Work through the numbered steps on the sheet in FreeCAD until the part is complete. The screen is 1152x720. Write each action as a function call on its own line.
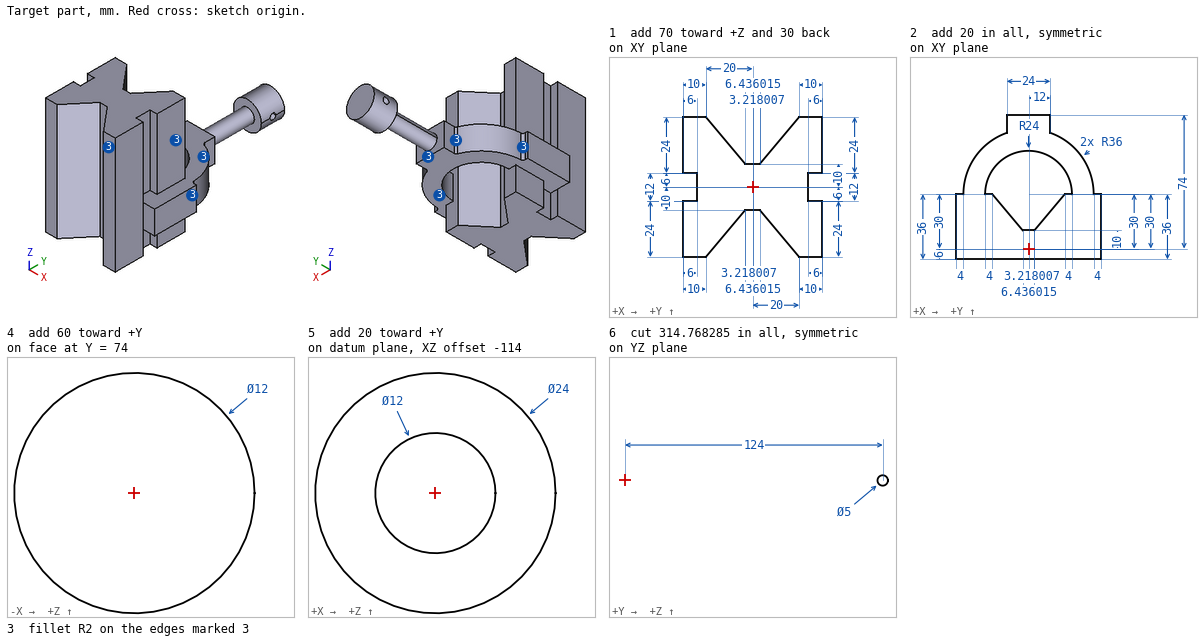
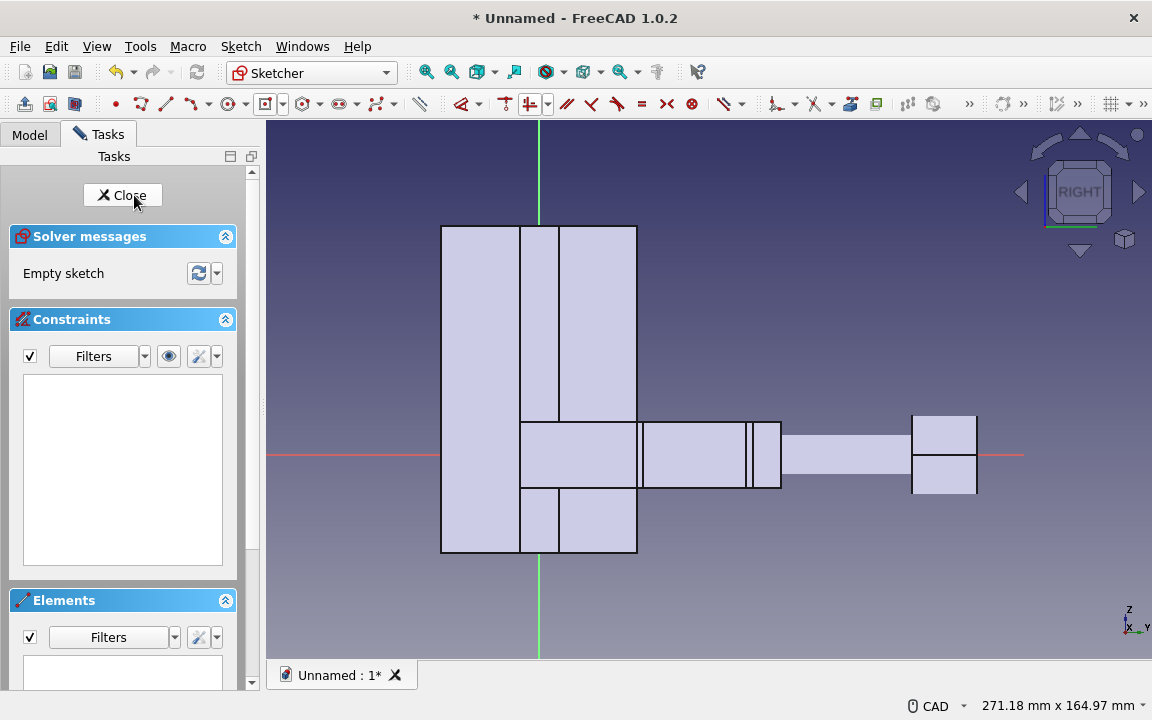
click(75, 104)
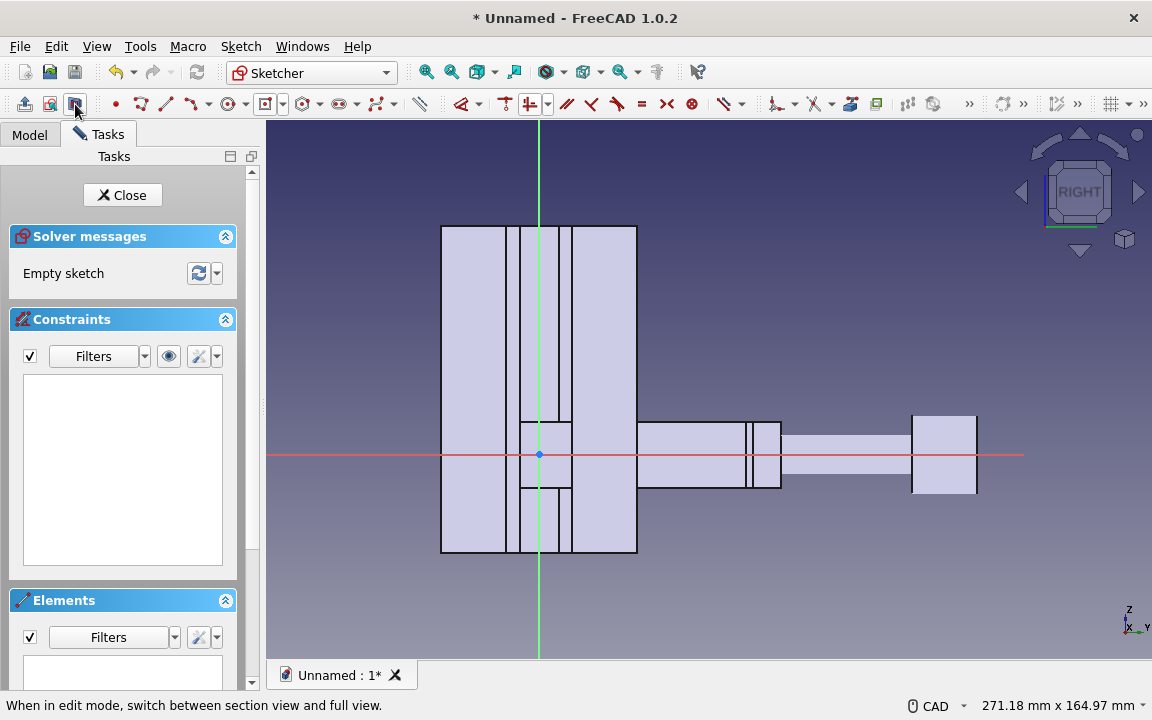
scroll(960, 458, up, 15)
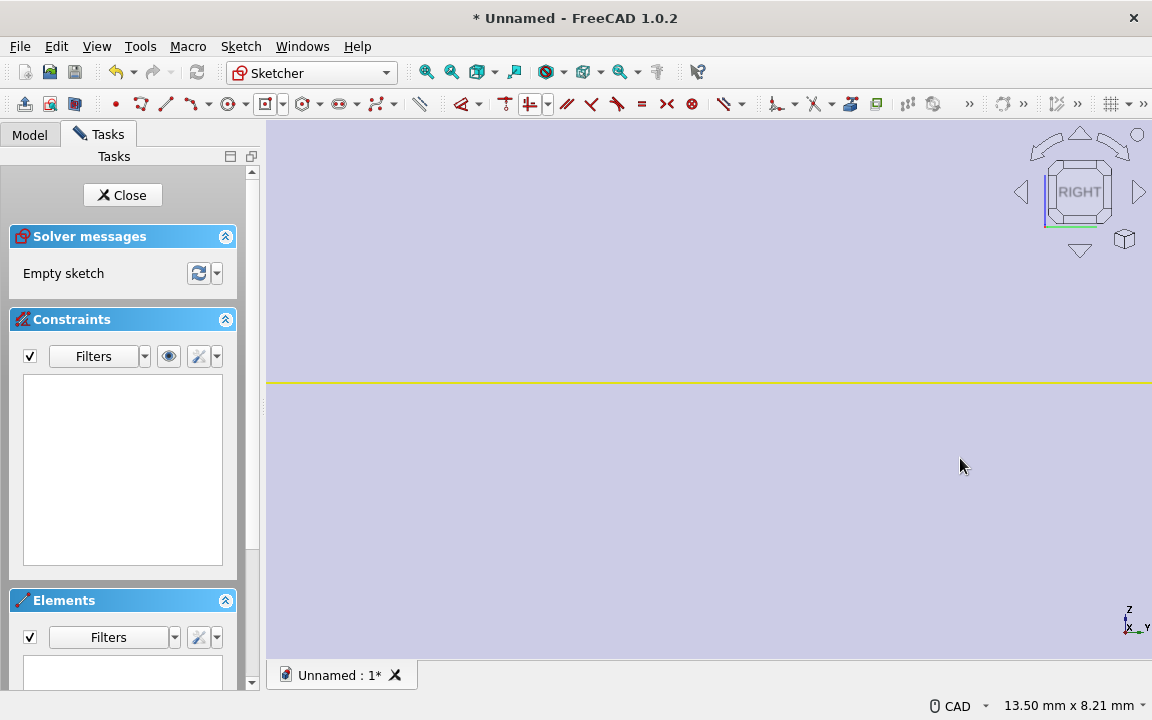
click(228, 104)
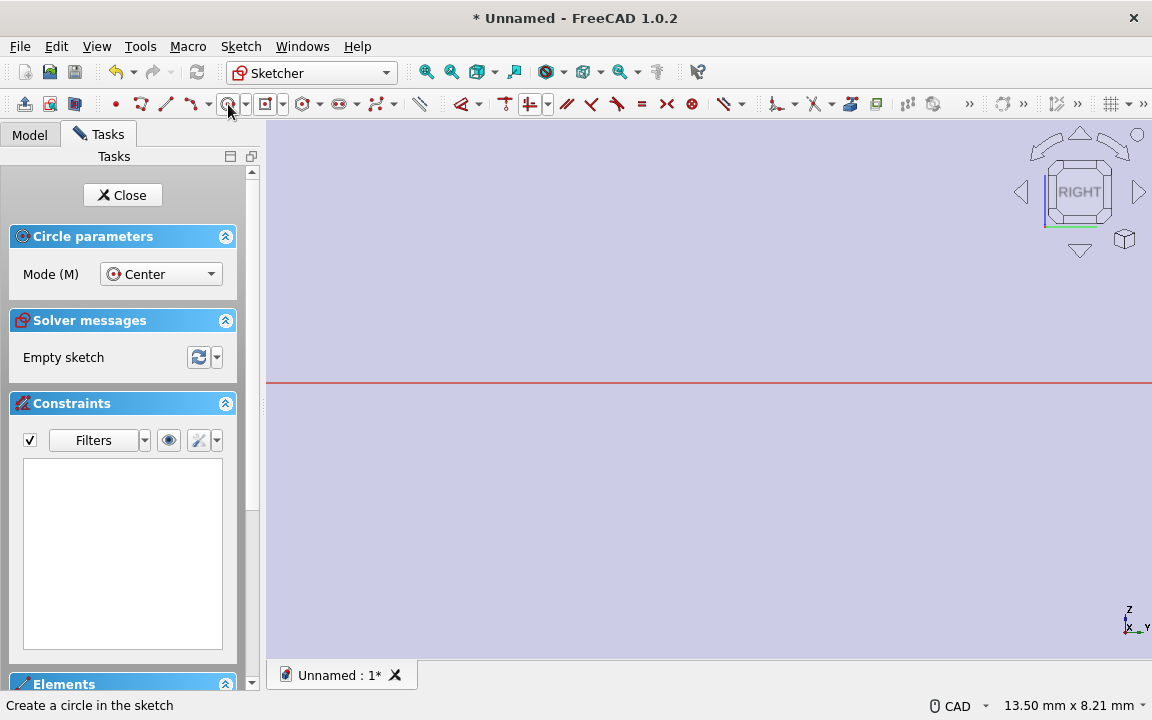
click(628, 383)
move(744, 267)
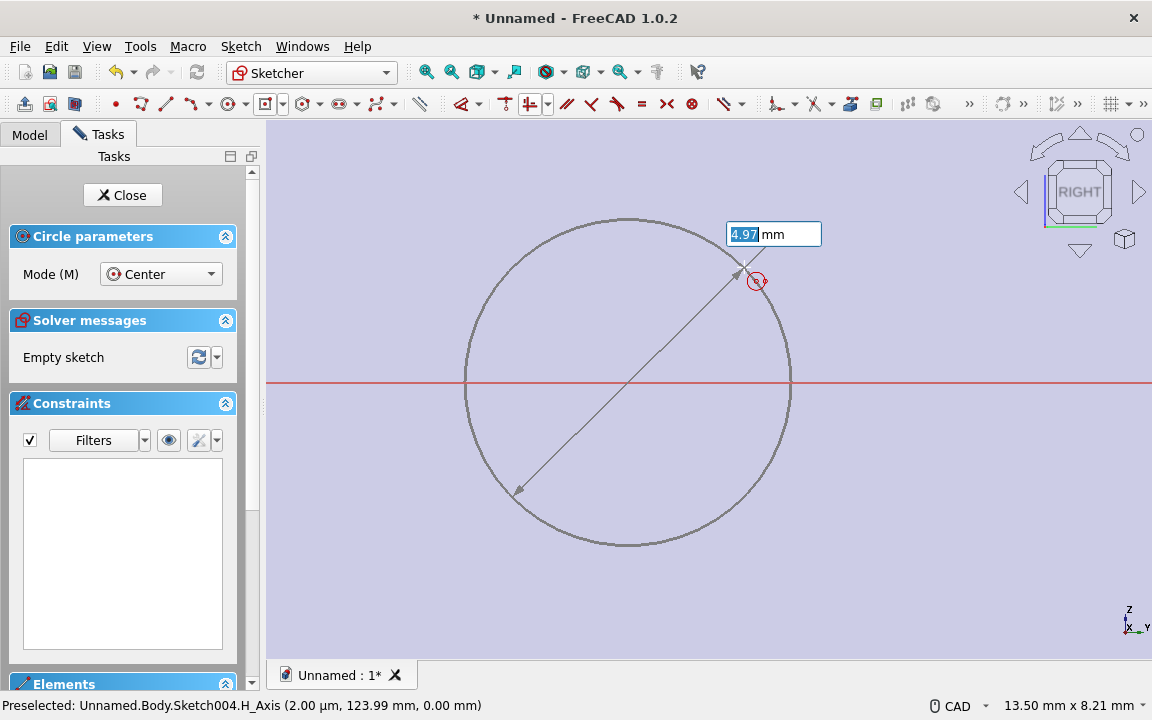
text(5)
key(Return)
key(Escape)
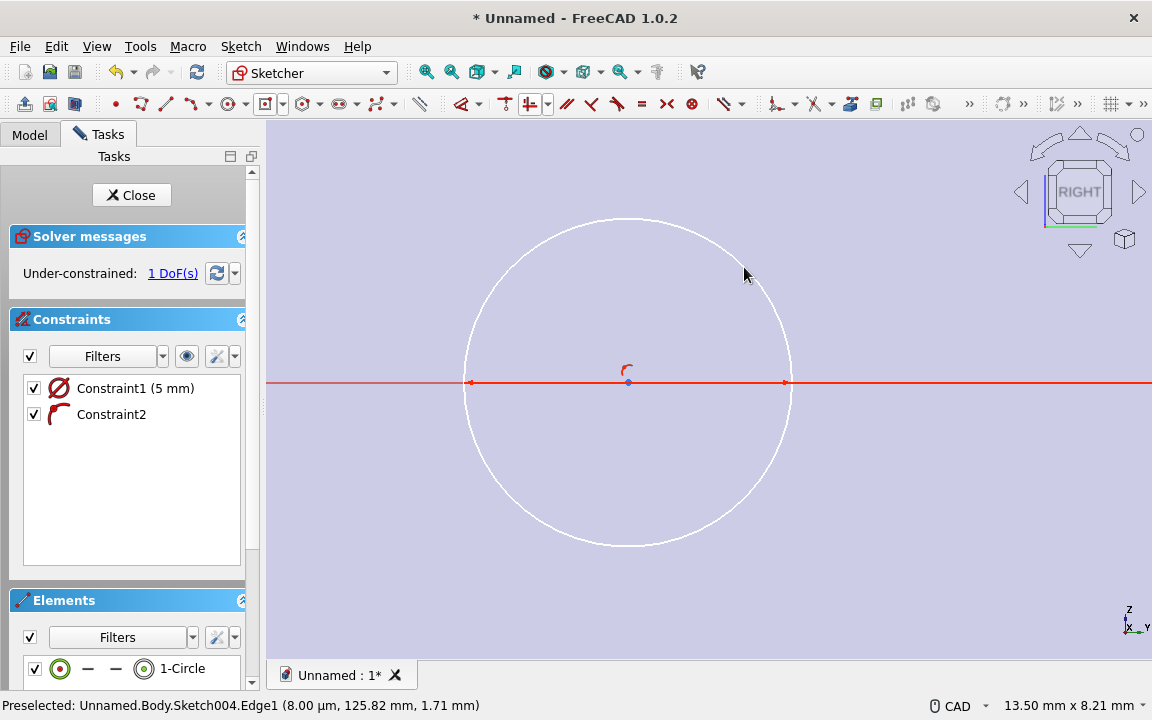
click(460, 104)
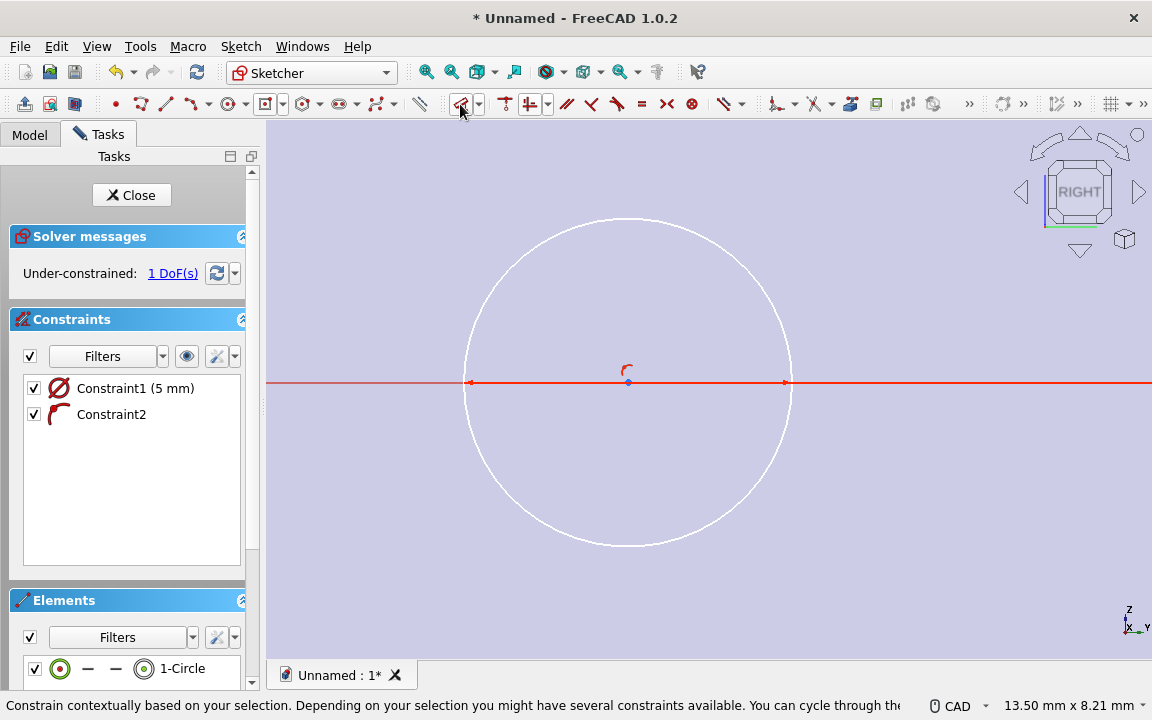
click(628, 383)
click(384, 417)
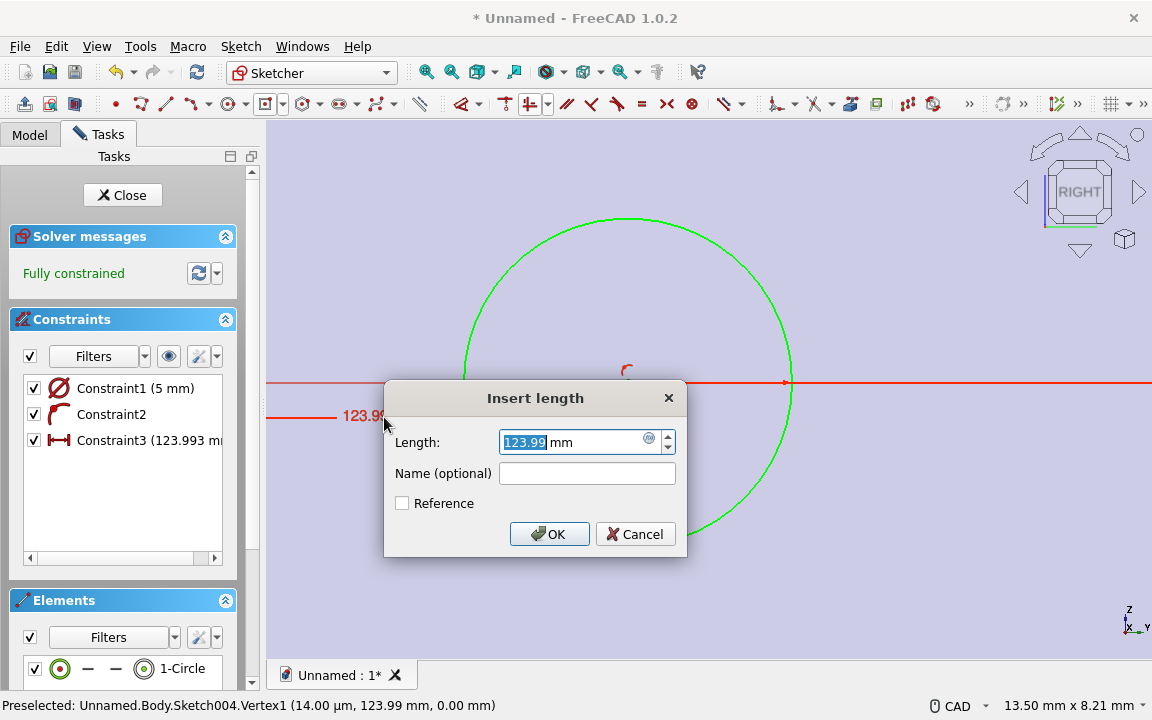
text(124)
key(Return)
key(Escape)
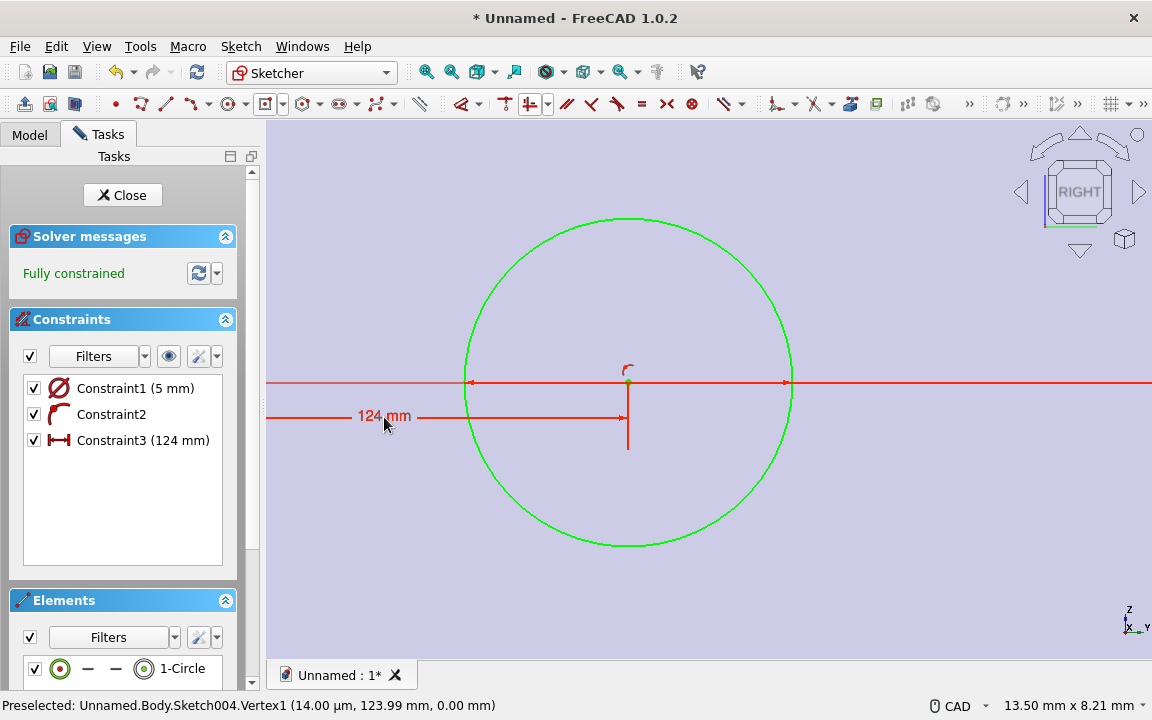
click(123, 195)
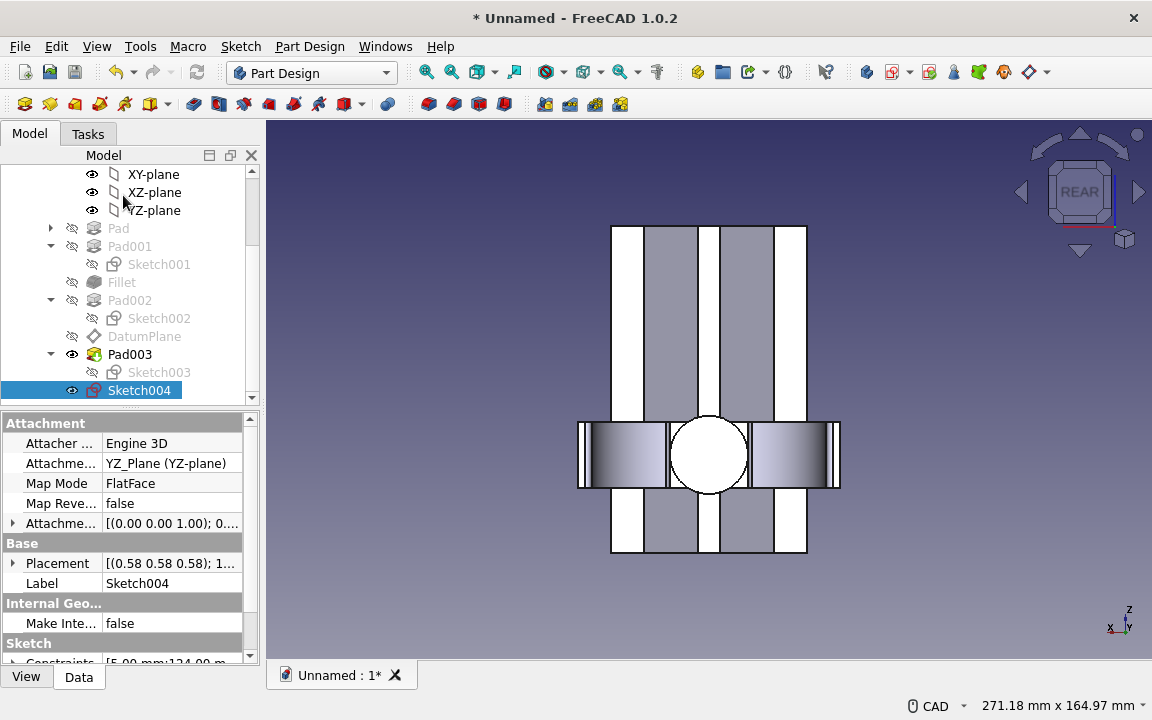
click(194, 104)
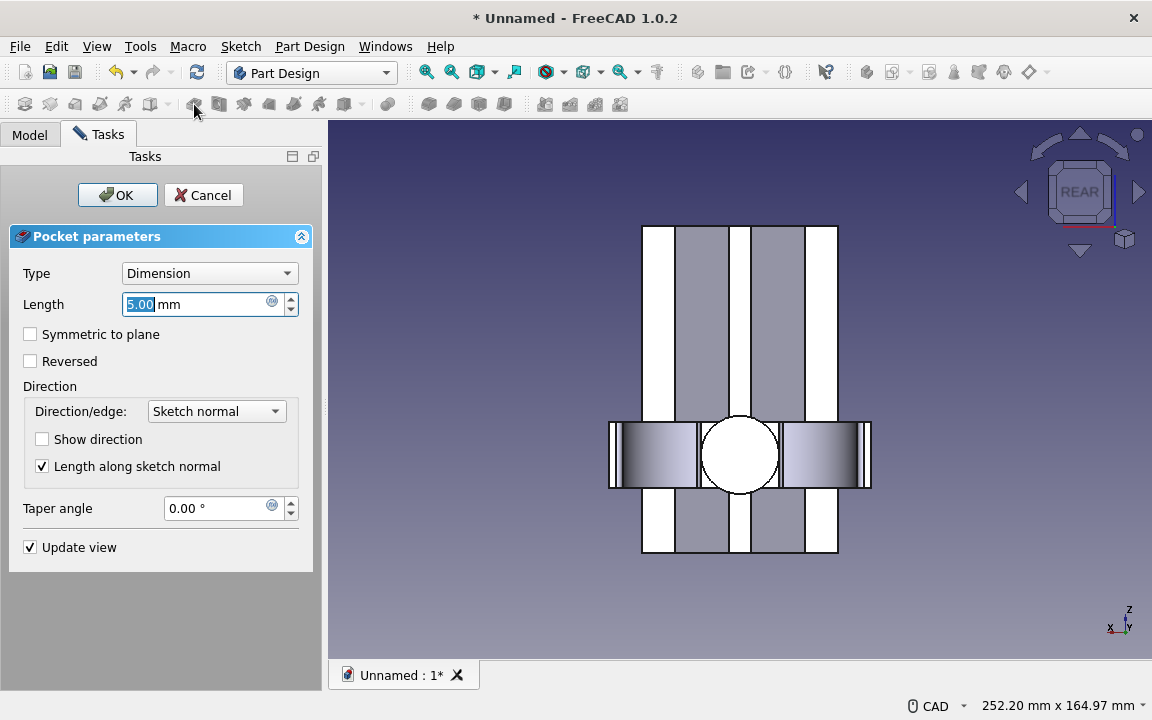
text(314.768285)
key(Tab)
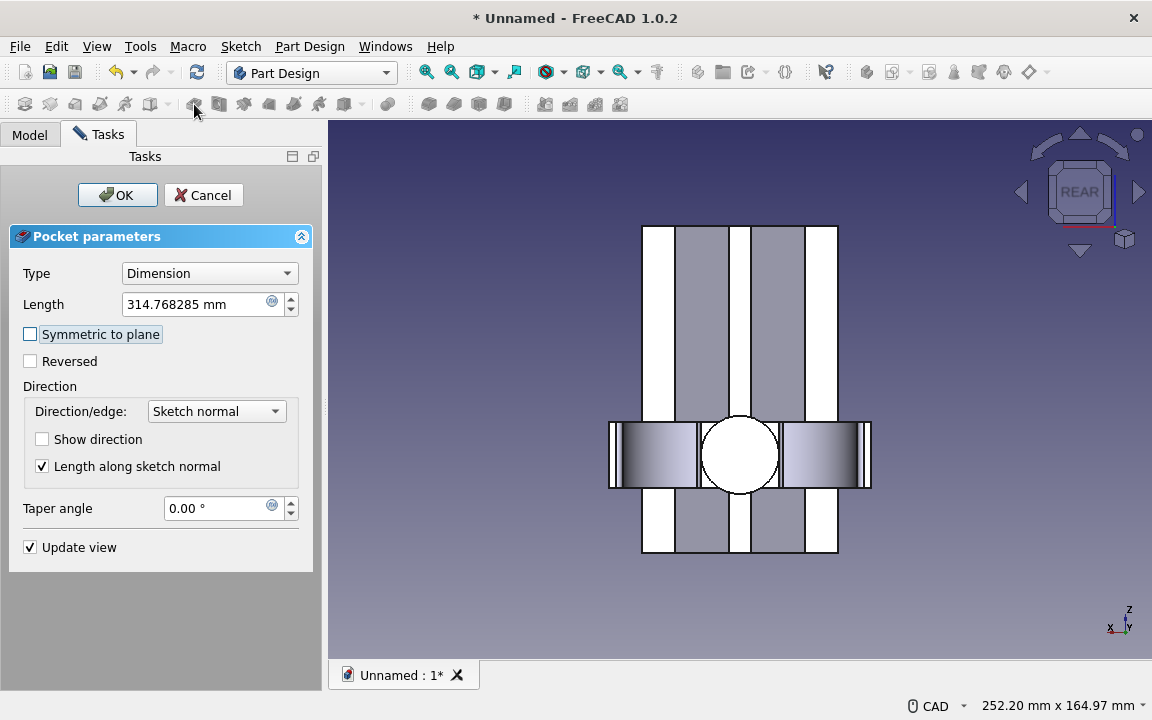
click(31, 334)